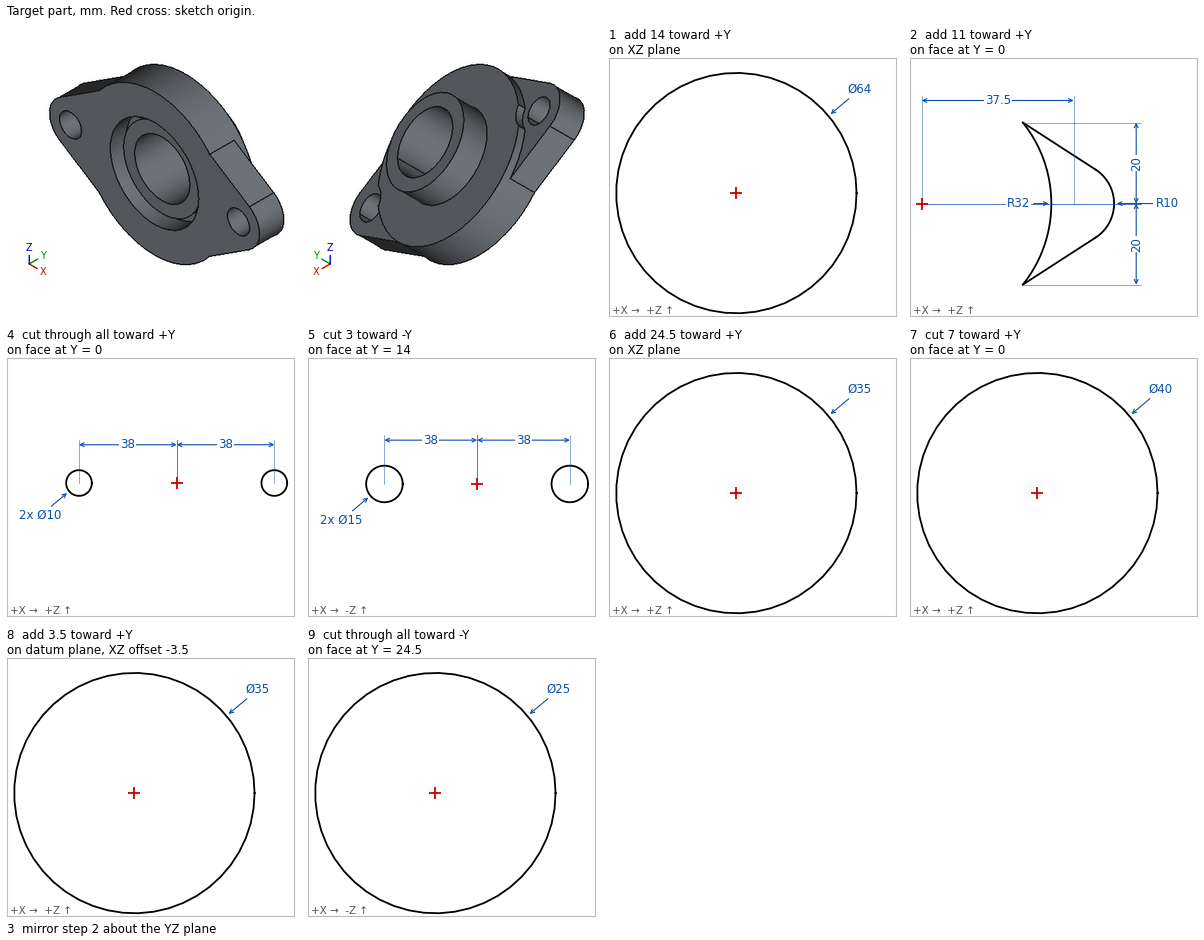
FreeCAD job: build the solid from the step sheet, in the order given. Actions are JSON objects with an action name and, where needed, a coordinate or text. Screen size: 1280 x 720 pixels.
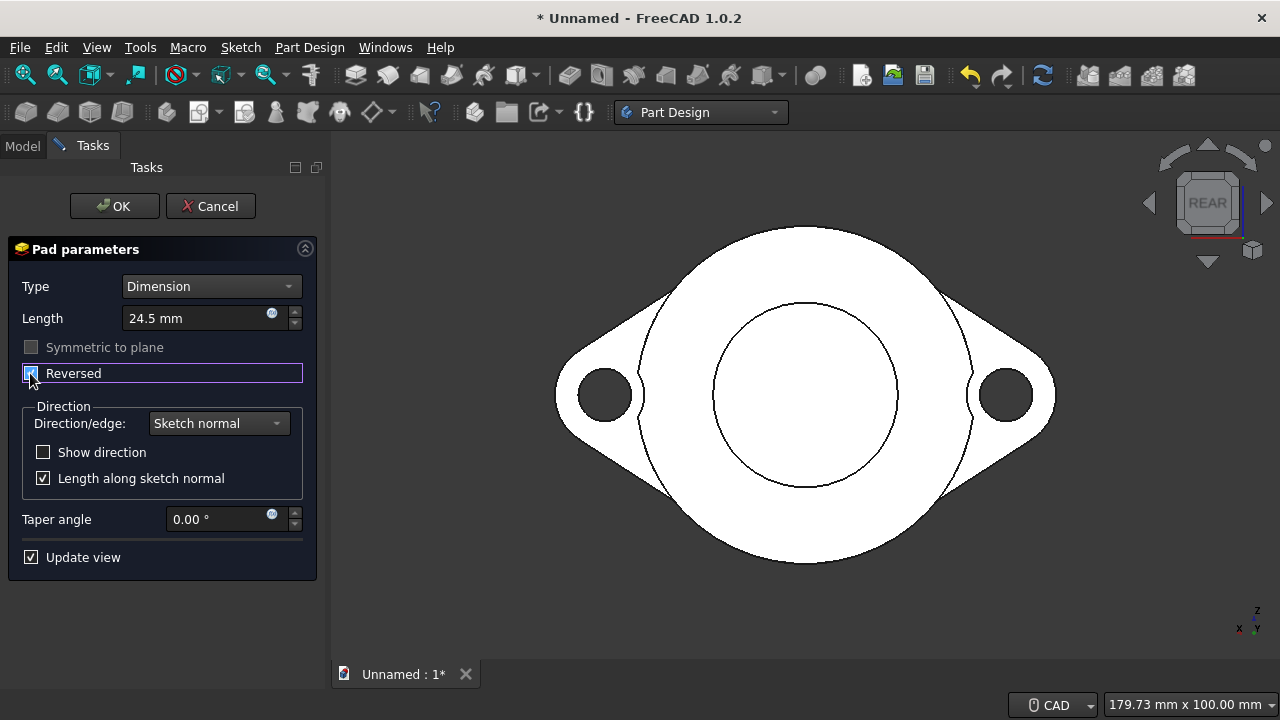
{"action": "left_click", "coordinate": [115, 206]}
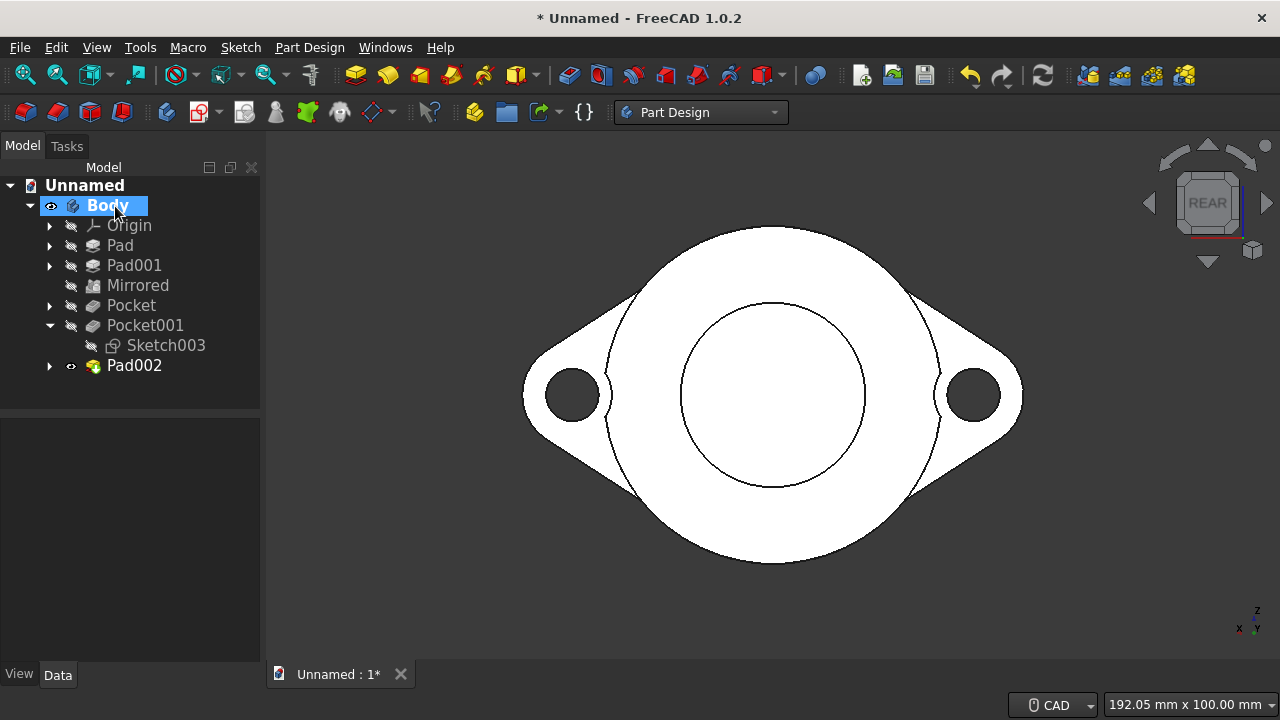
{"action": "key", "text": "0"}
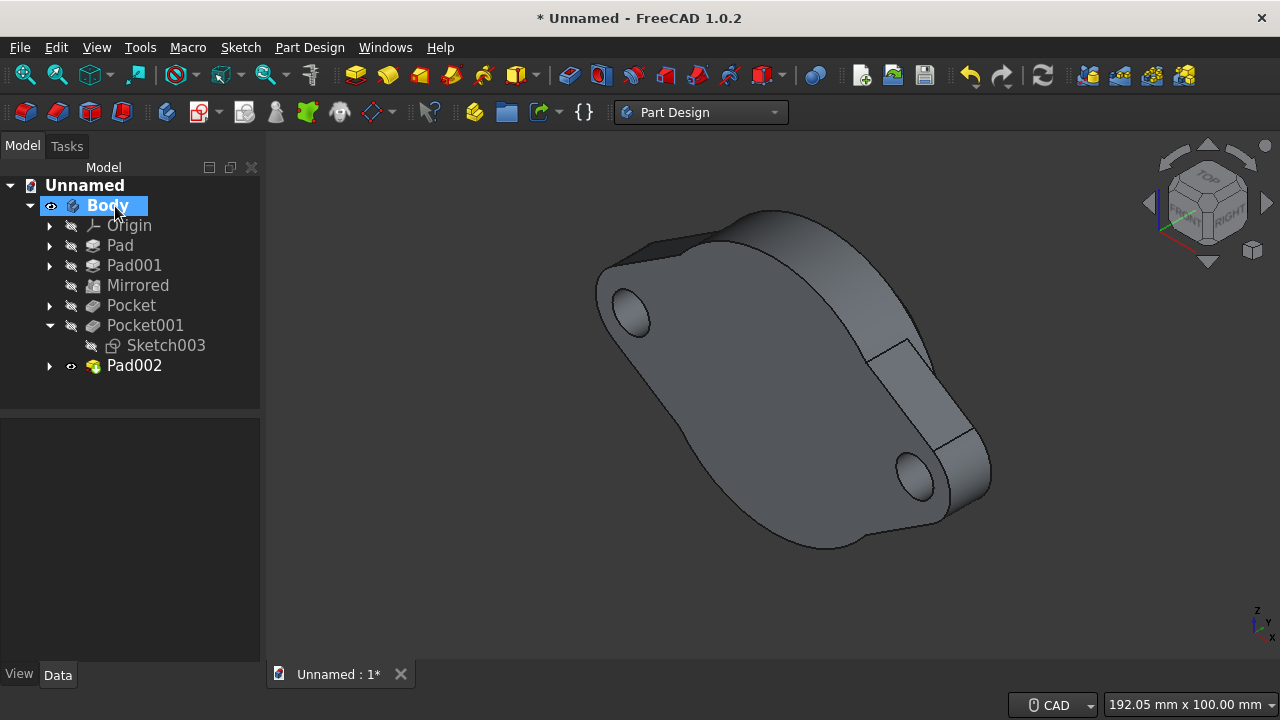
{"action": "key", "text": "v f"}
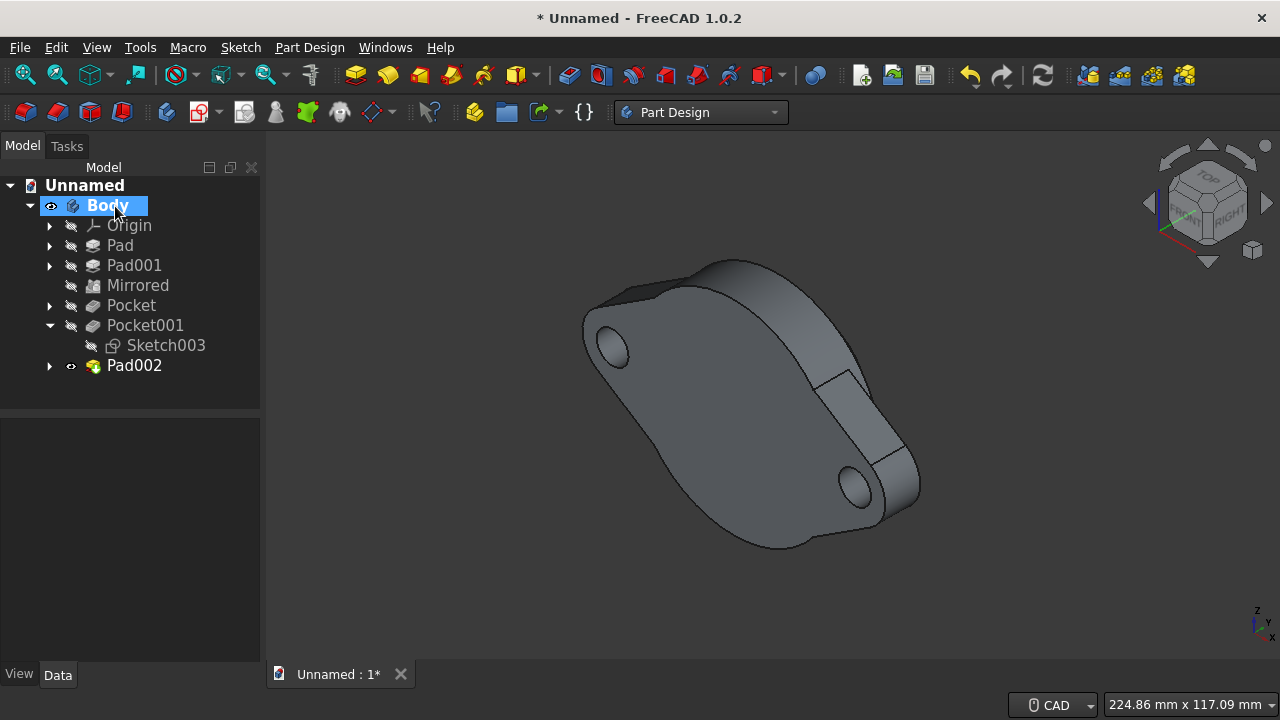
{"action": "left_click", "coordinate": [734, 416]}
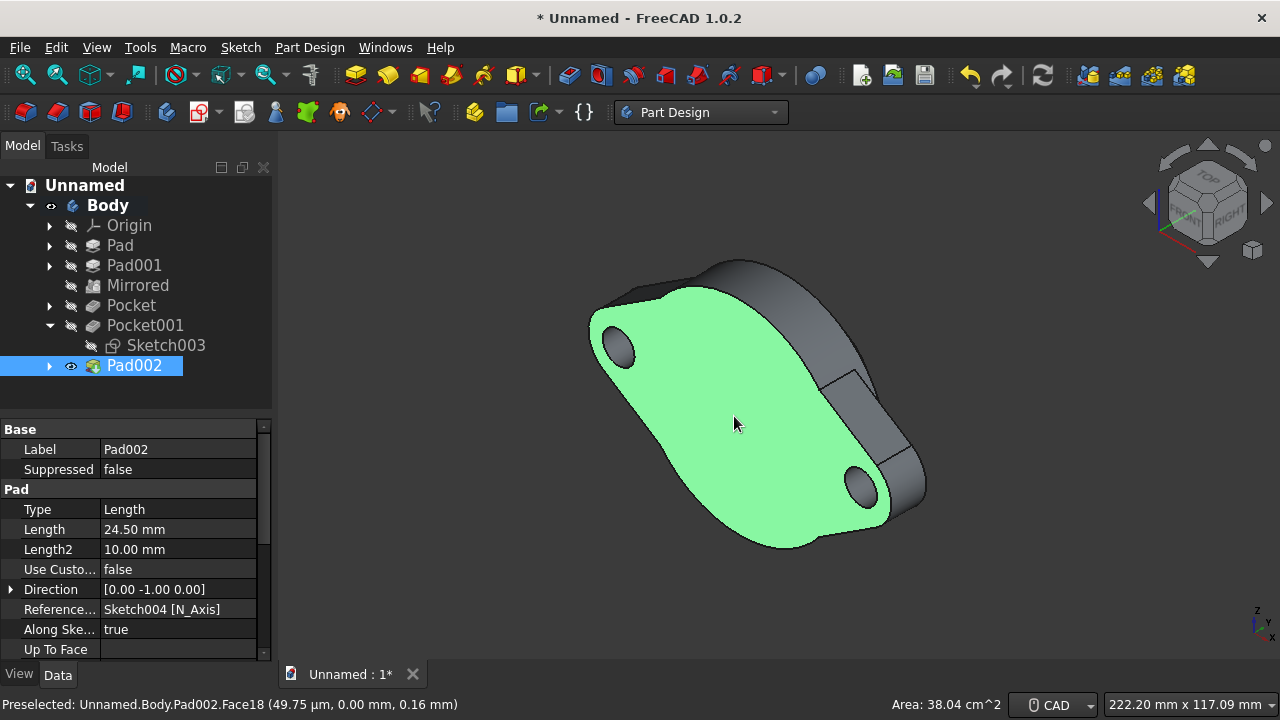
{"action": "left_click", "coordinate": [200, 112]}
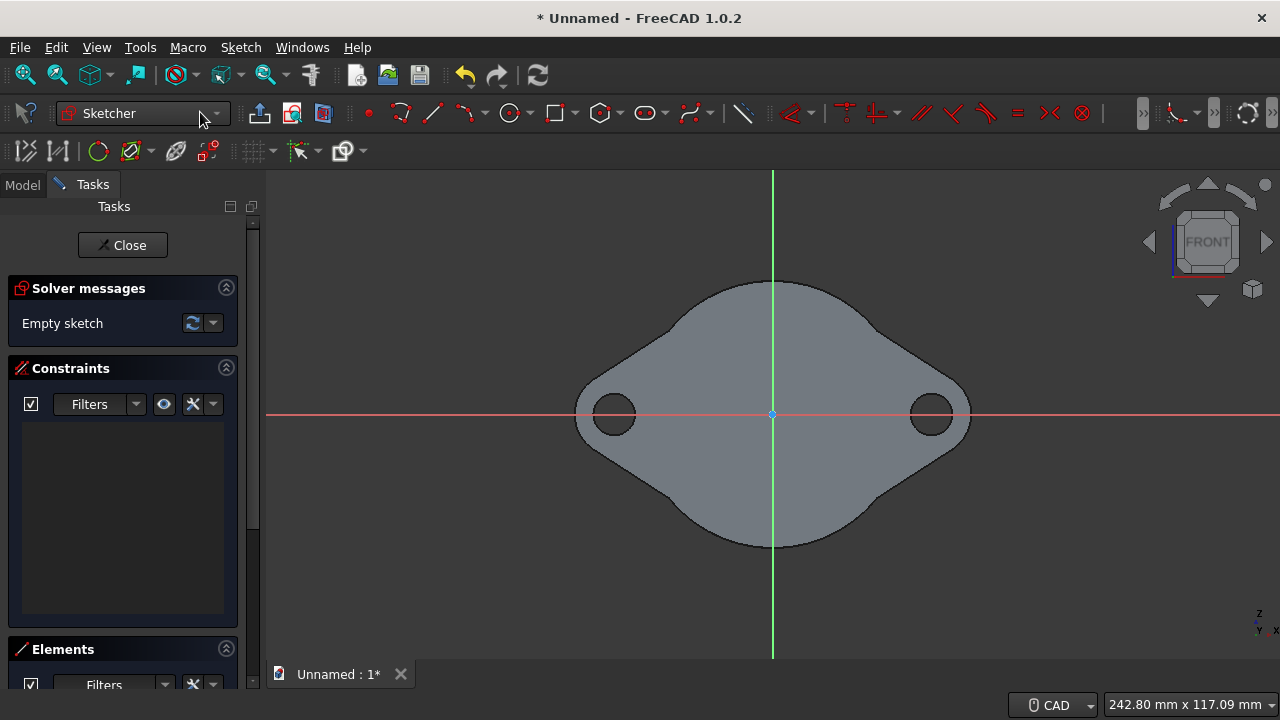
{"action": "scroll", "coordinate": [856, 415], "scroll_direction": "up", "scroll_amount": 3}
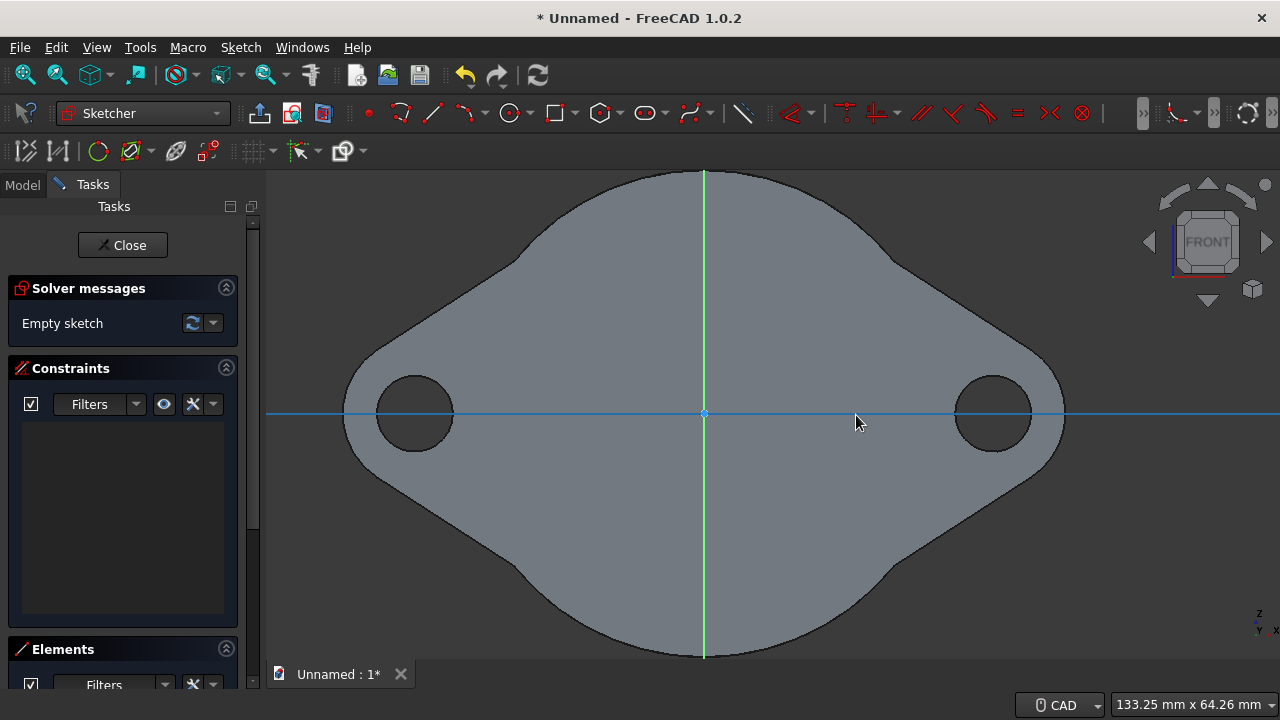
{"action": "left_click", "coordinate": [510, 114]}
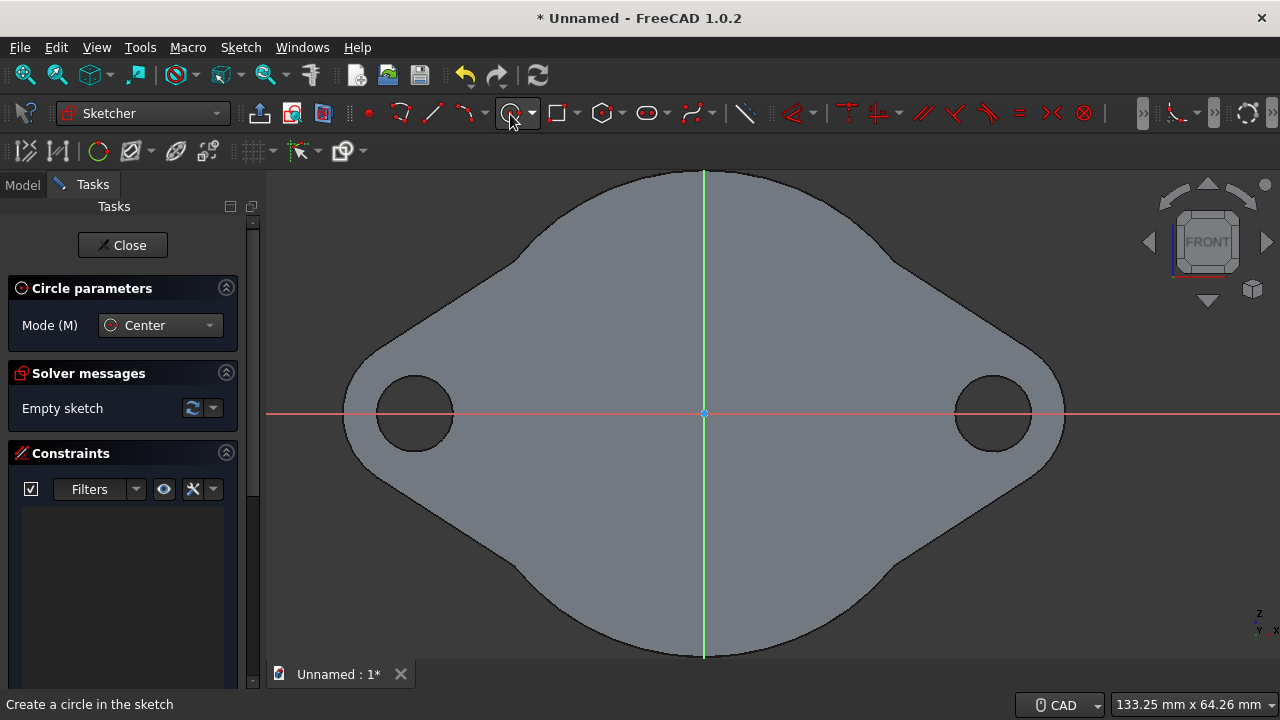
{"action": "left_click", "coordinate": [704, 414]}
{"action": "left_click", "coordinate": [812, 306]}
{"action": "key", "text": "Escape"}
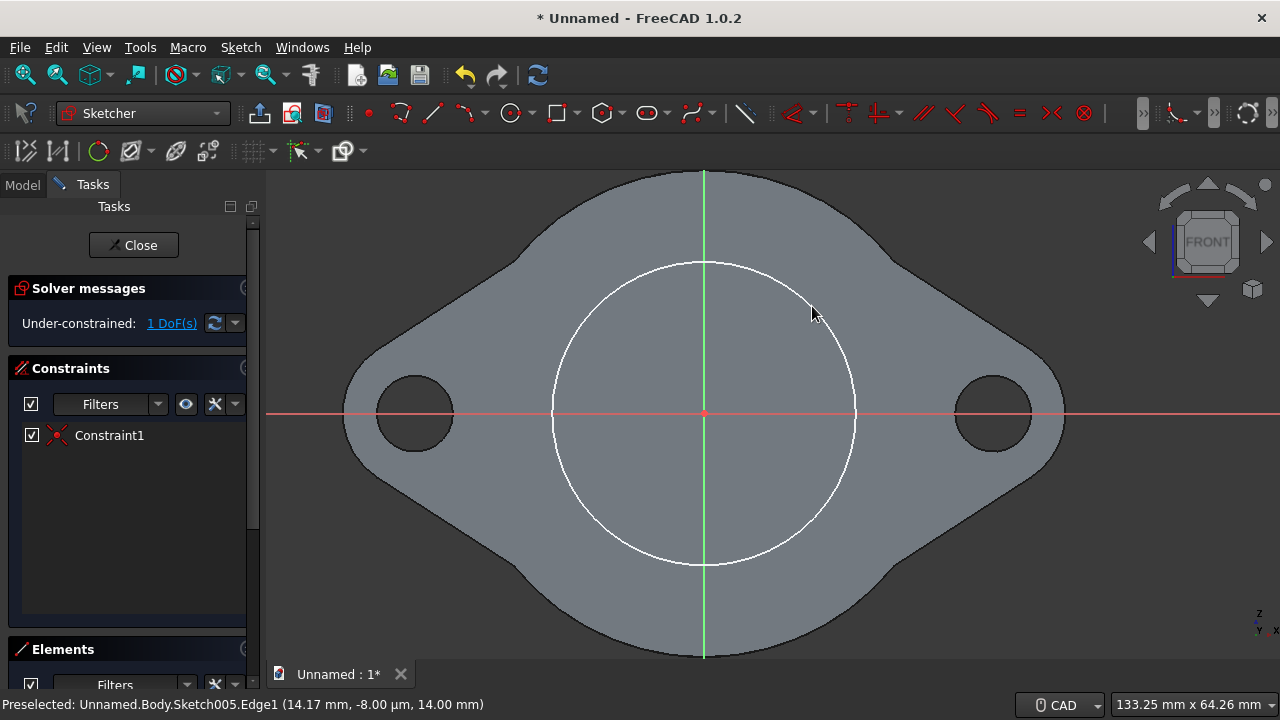
{"action": "left_click", "coordinate": [792, 114]}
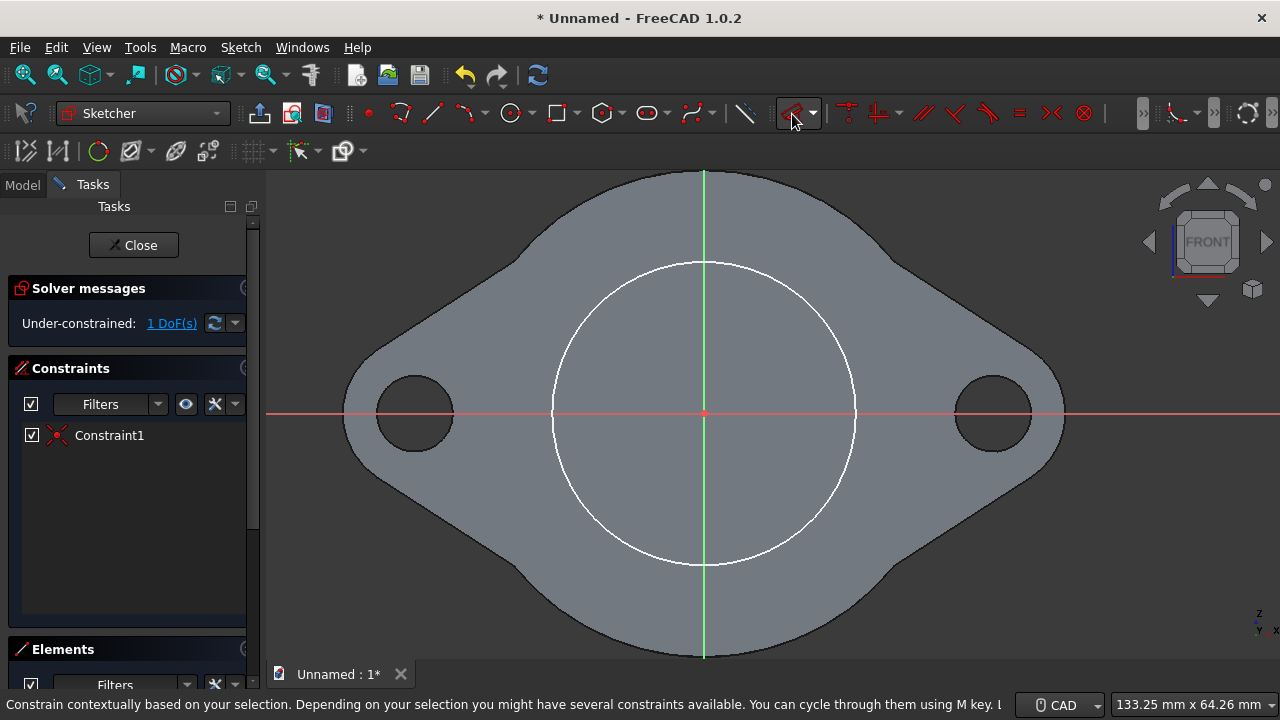
{"action": "left_click", "coordinate": [811, 306]}
{"action": "left_click", "coordinate": [834, 283]}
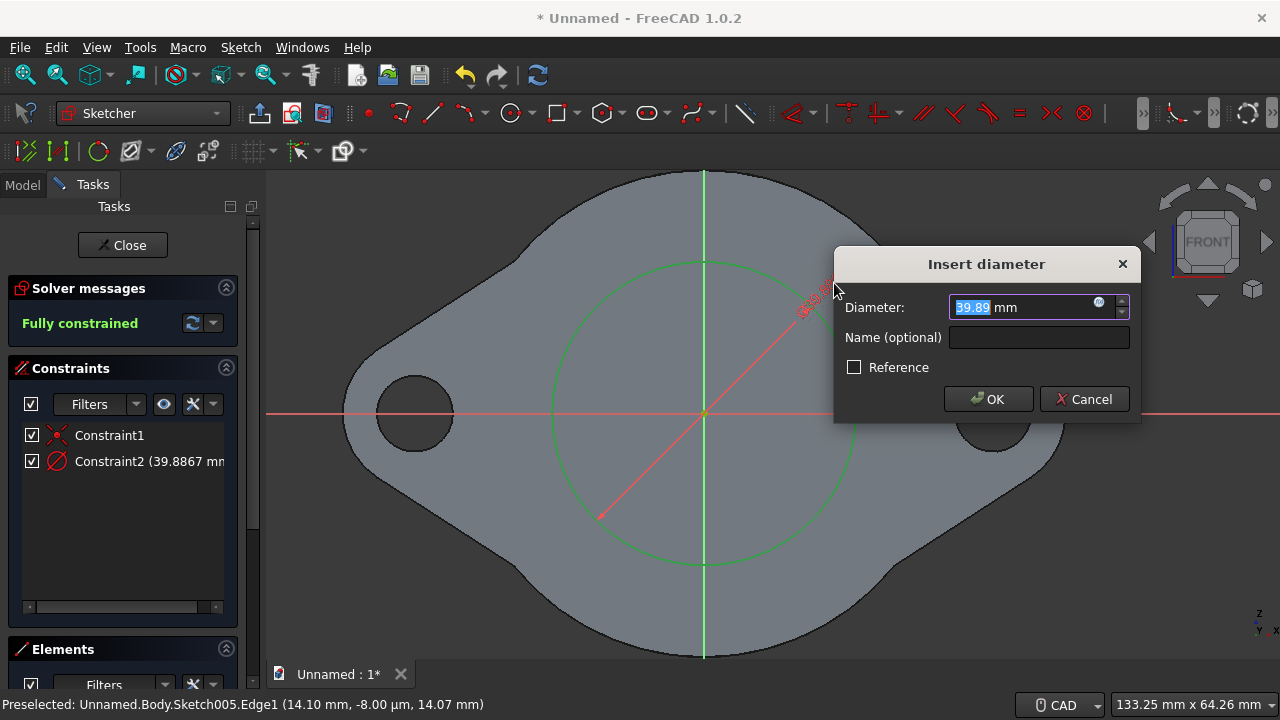
{"action": "type", "text": "40"}
{"action": "key", "text": "Return"}
{"action": "key", "text": "Escape"}